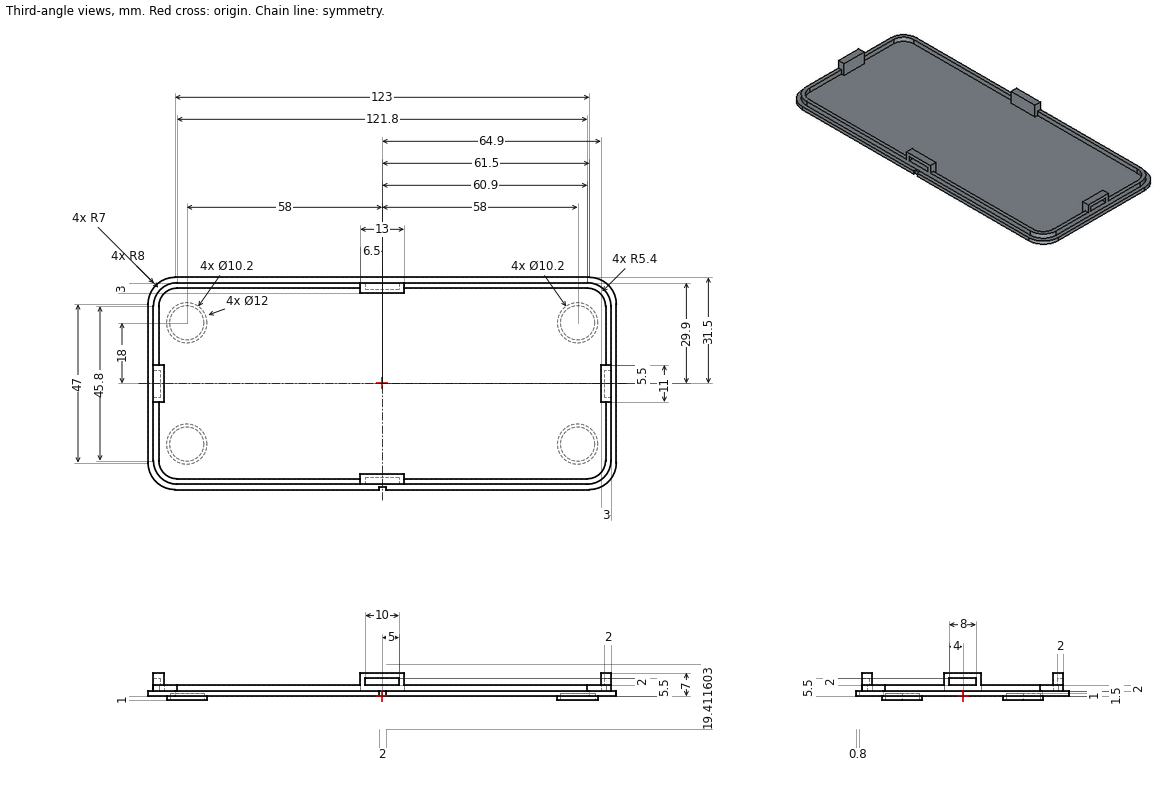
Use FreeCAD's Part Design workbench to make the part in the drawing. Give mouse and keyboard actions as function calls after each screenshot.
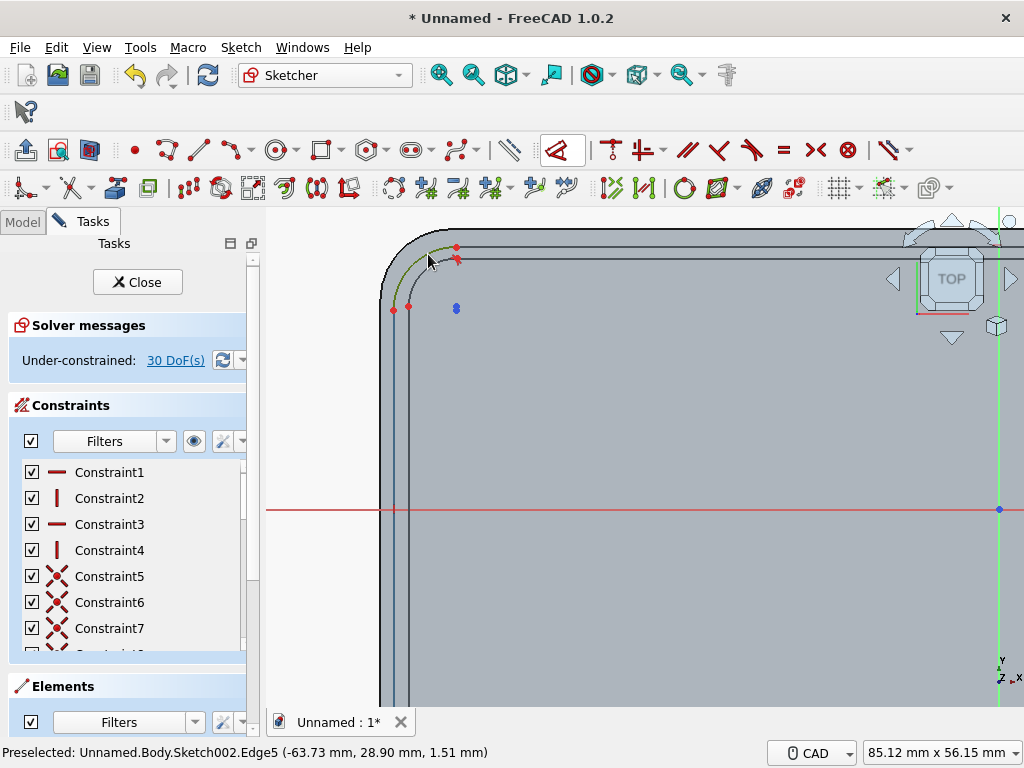
click(752, 150)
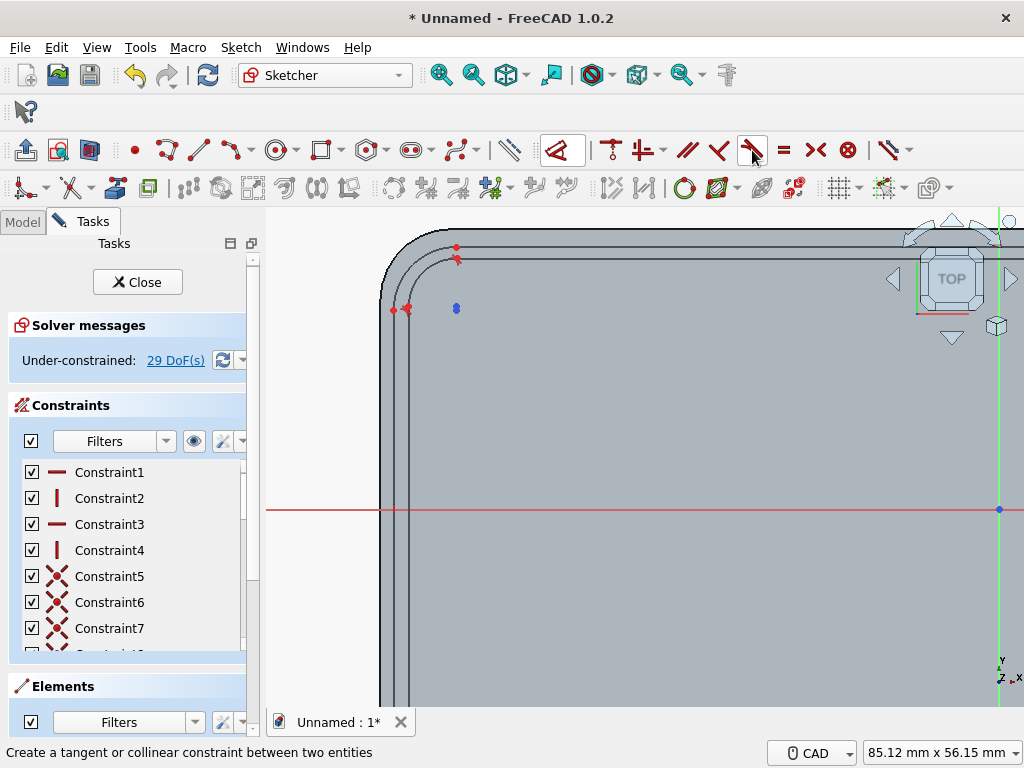
click(394, 433)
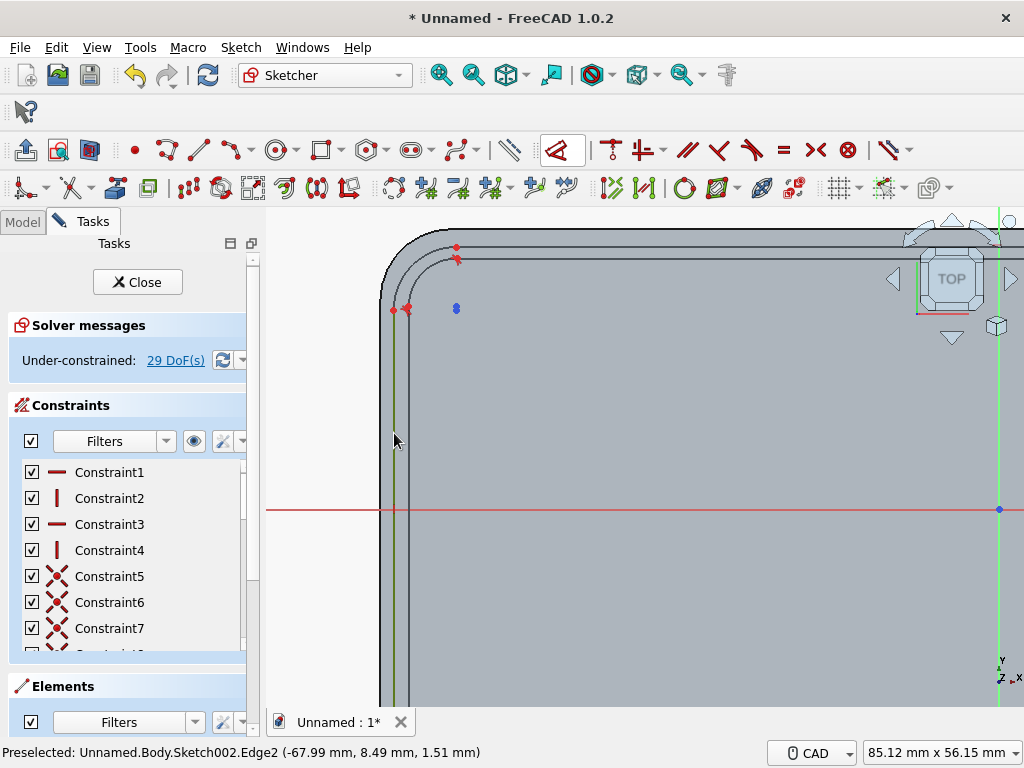
scroll(394, 434, down, 6)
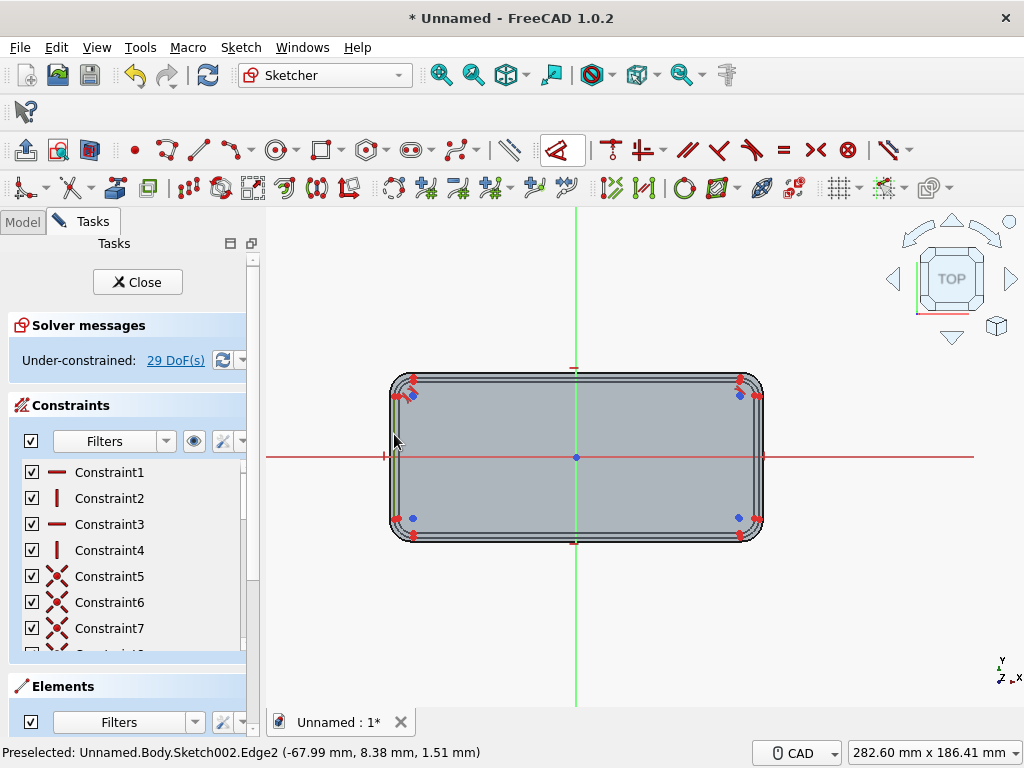
scroll(397, 528, up, 6)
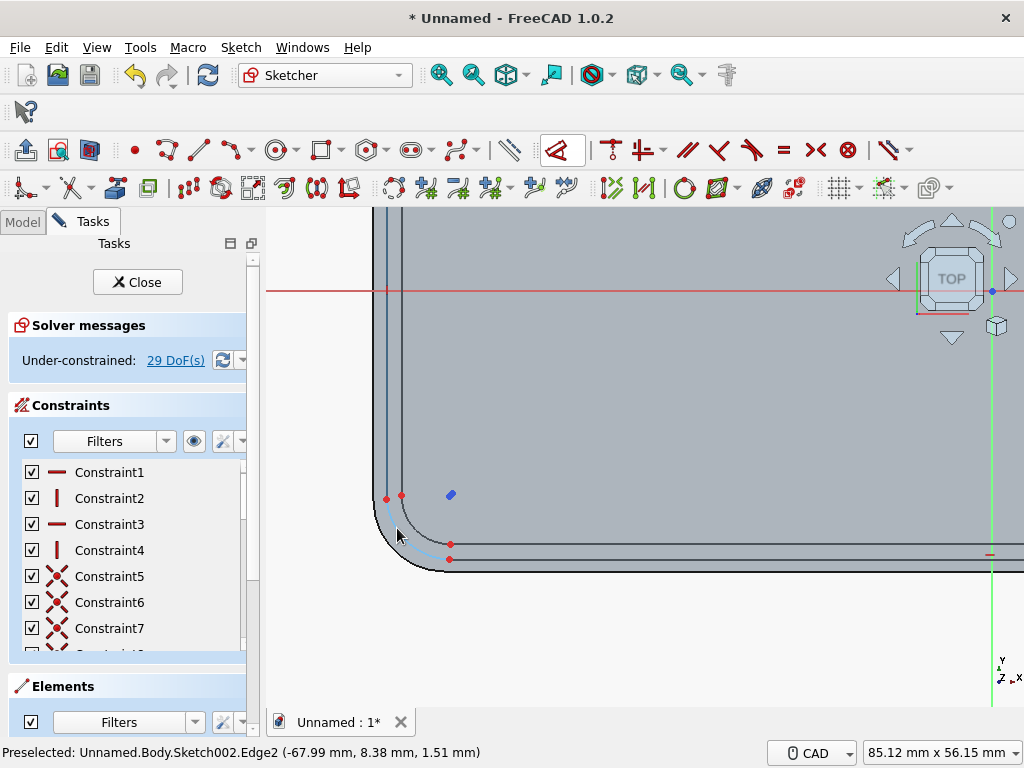
click(395, 527)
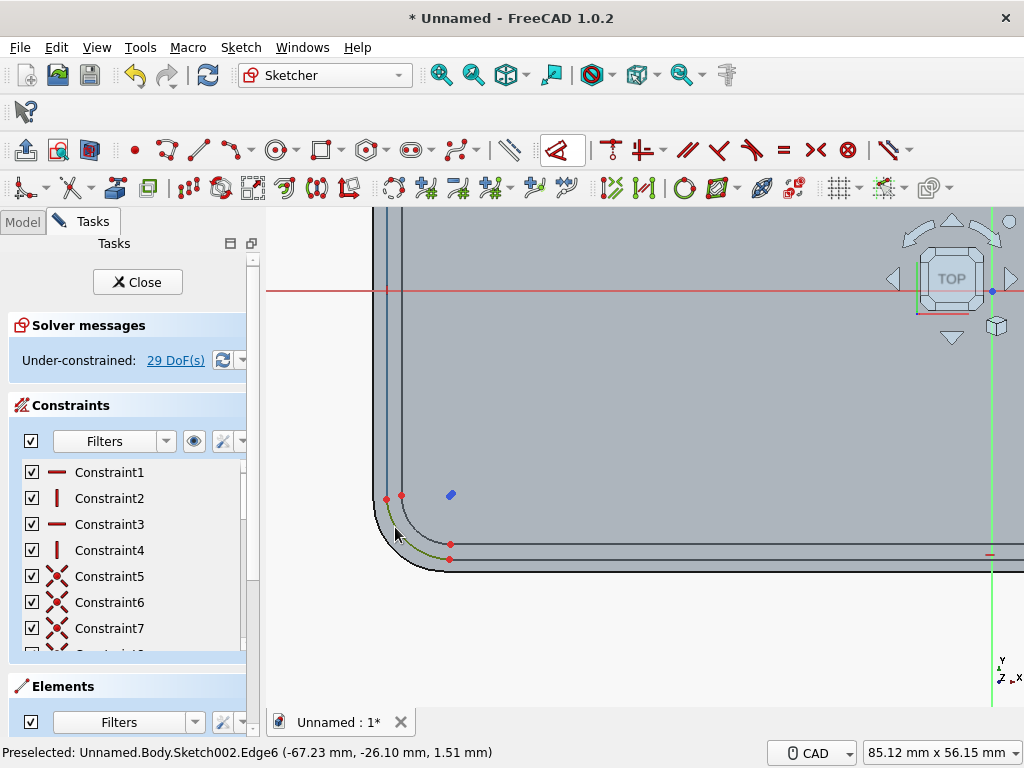
click(752, 150)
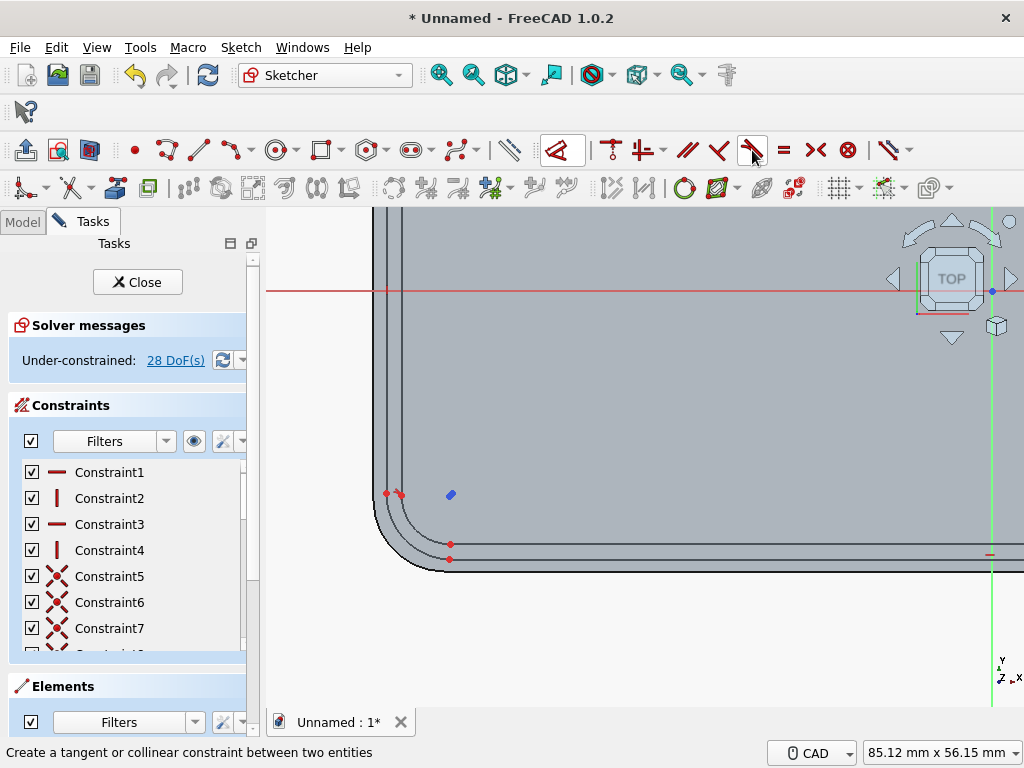
click(776, 560)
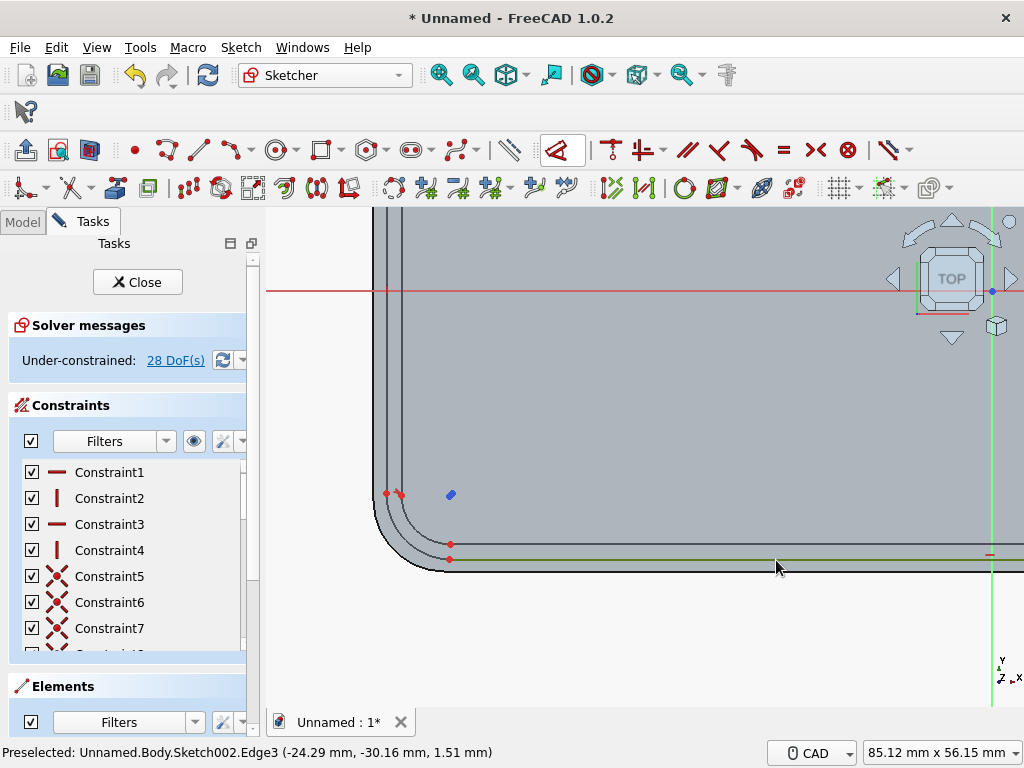
click(393, 523)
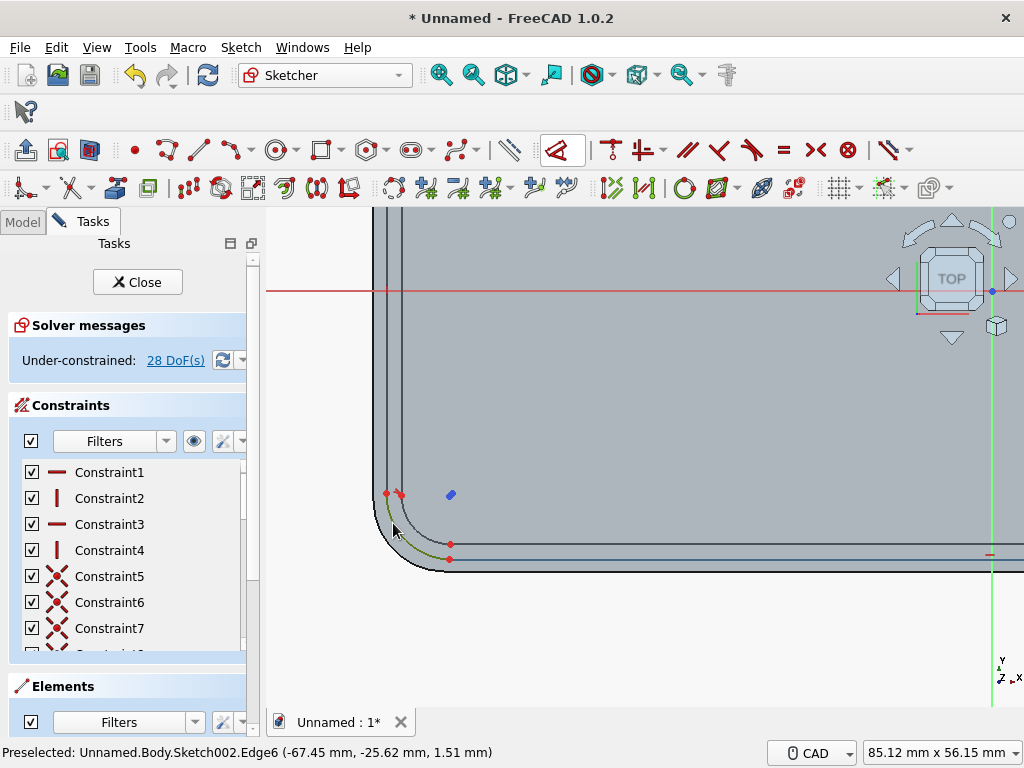
key(t)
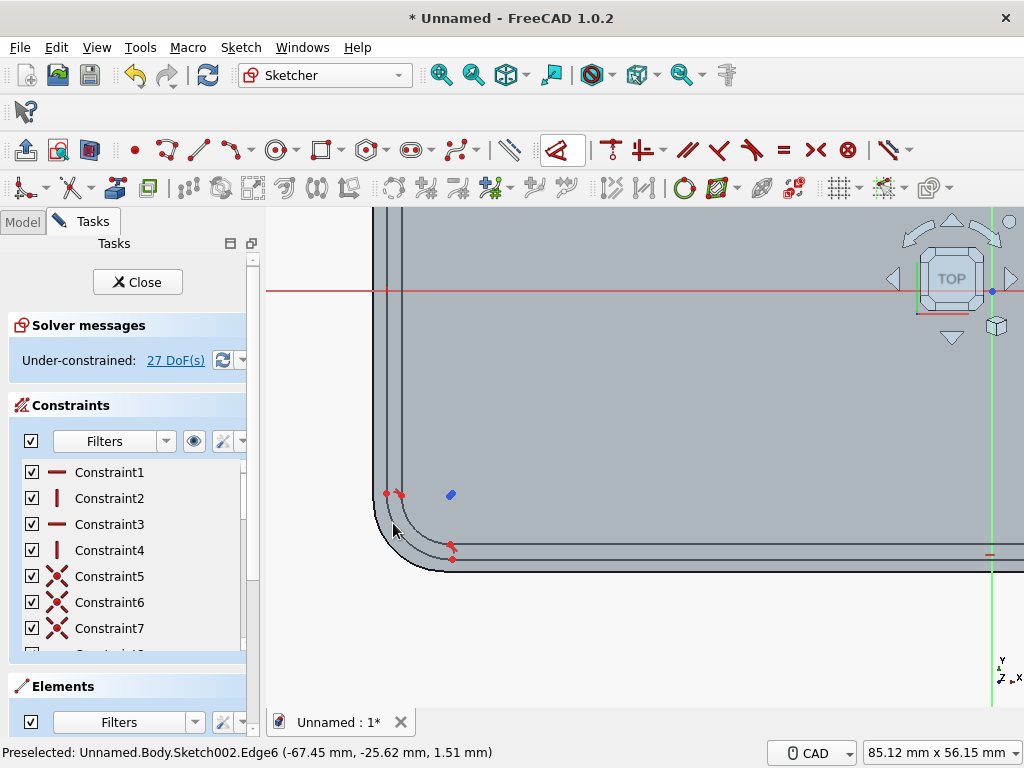
click(778, 560)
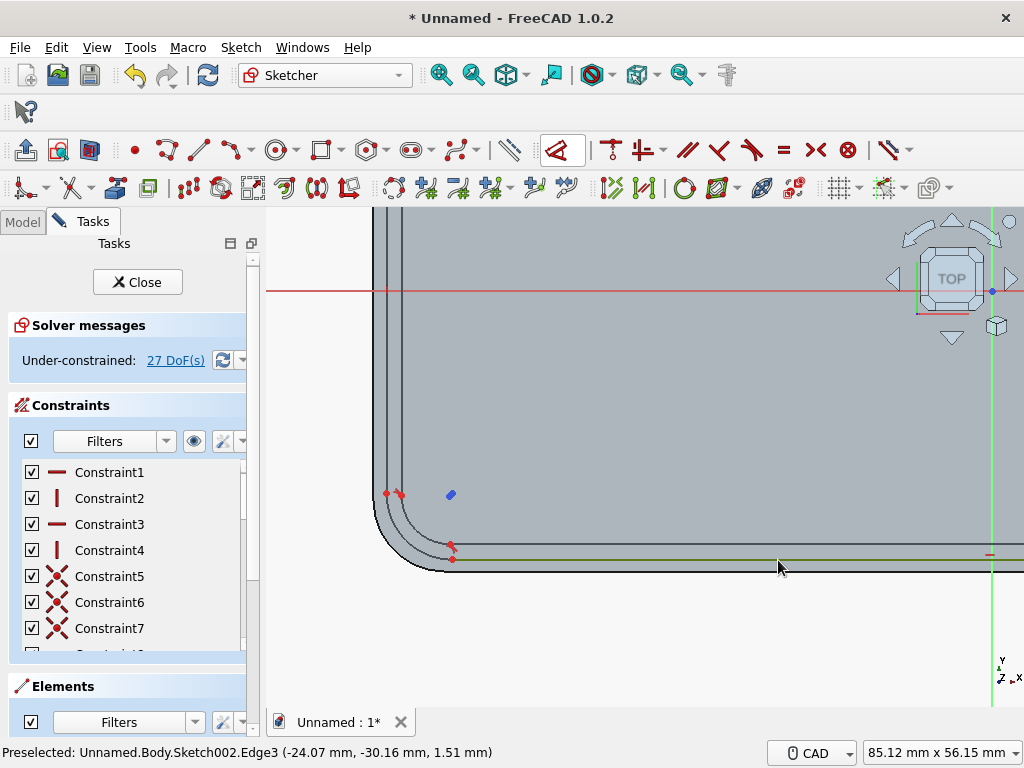
scroll(397, 529, down, 6)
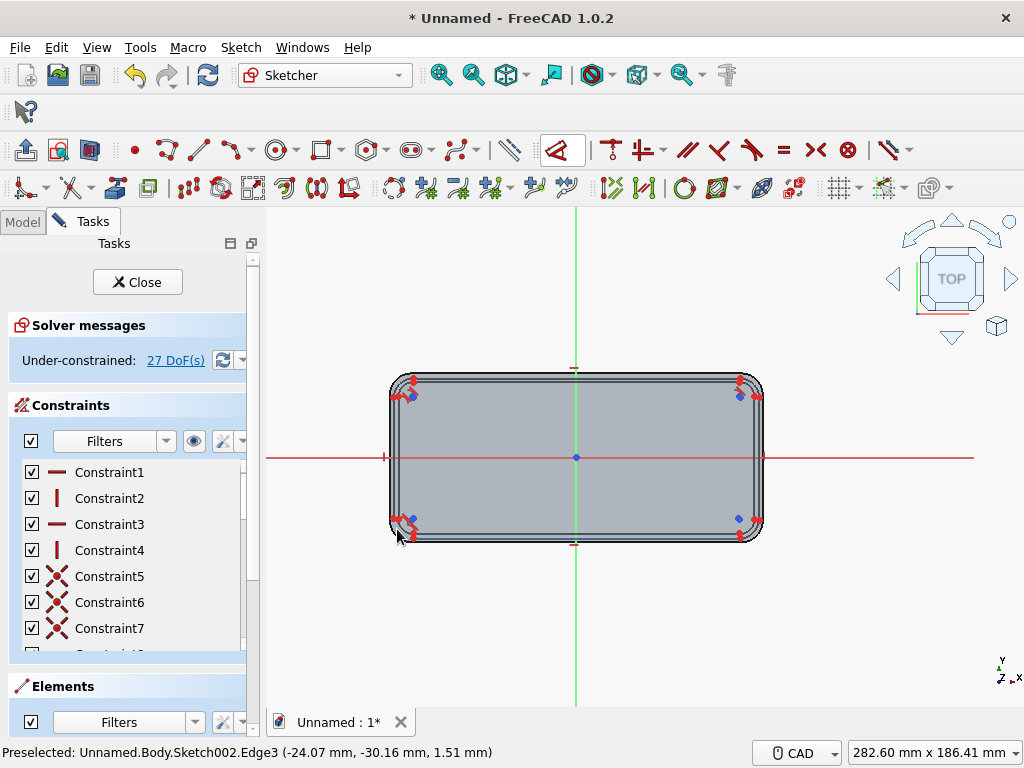
scroll(748, 536, up, 6)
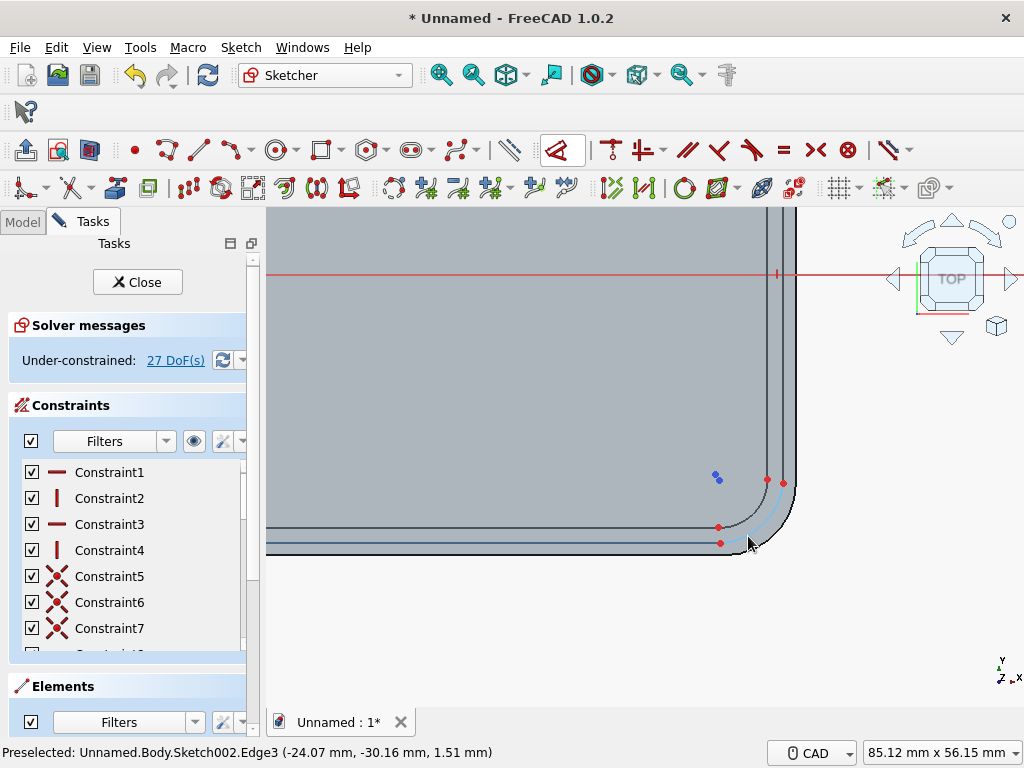
click(747, 536)